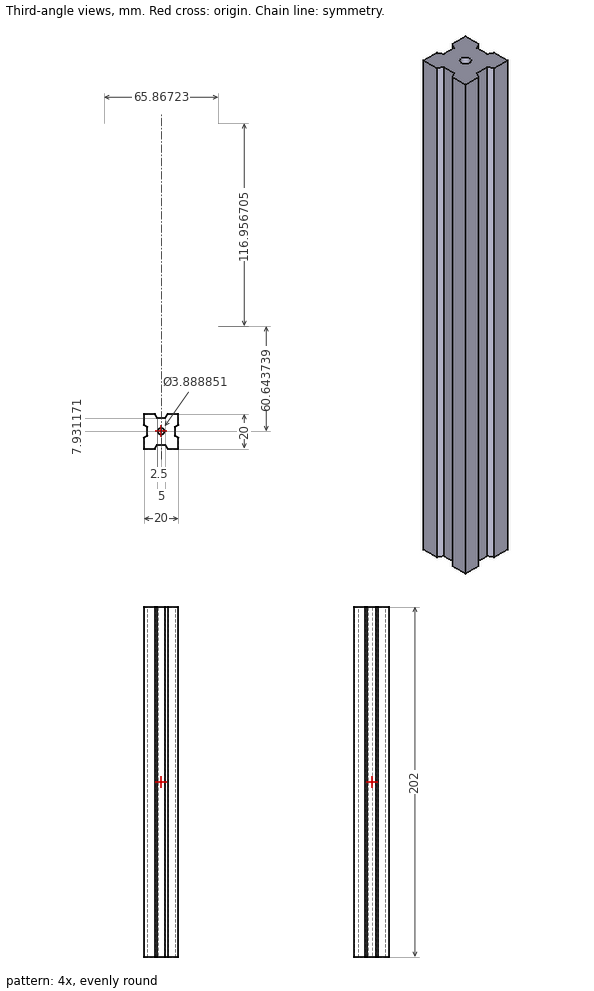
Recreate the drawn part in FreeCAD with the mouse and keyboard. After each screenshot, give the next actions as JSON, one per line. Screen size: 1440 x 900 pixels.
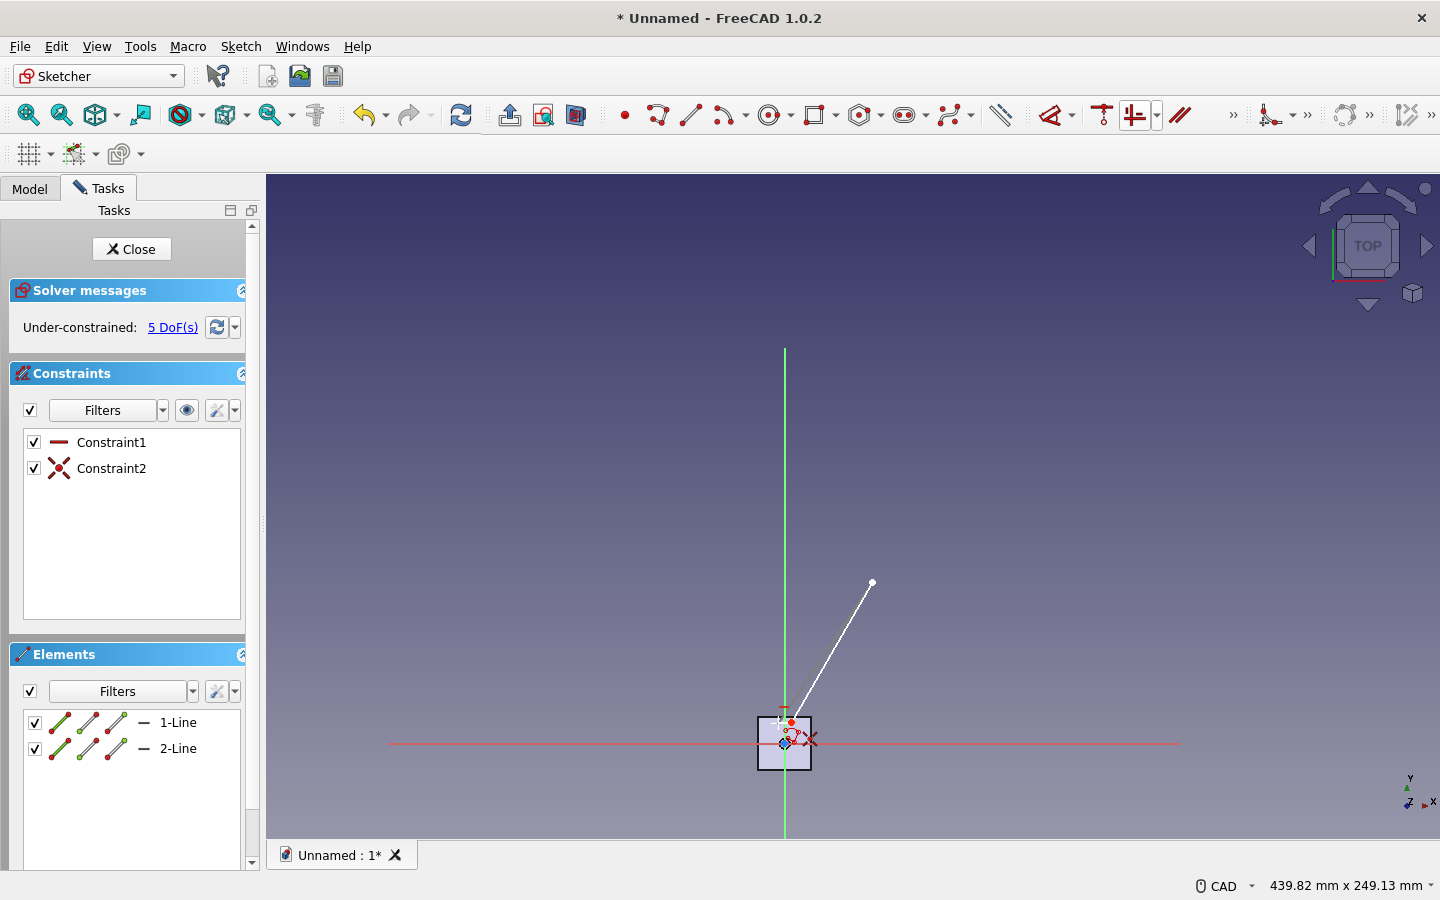
{"action": "left_click", "coordinate": [873, 270]}
{"action": "left_click", "coordinate": [697, 270]}
{"action": "left_click", "coordinate": [697, 582]}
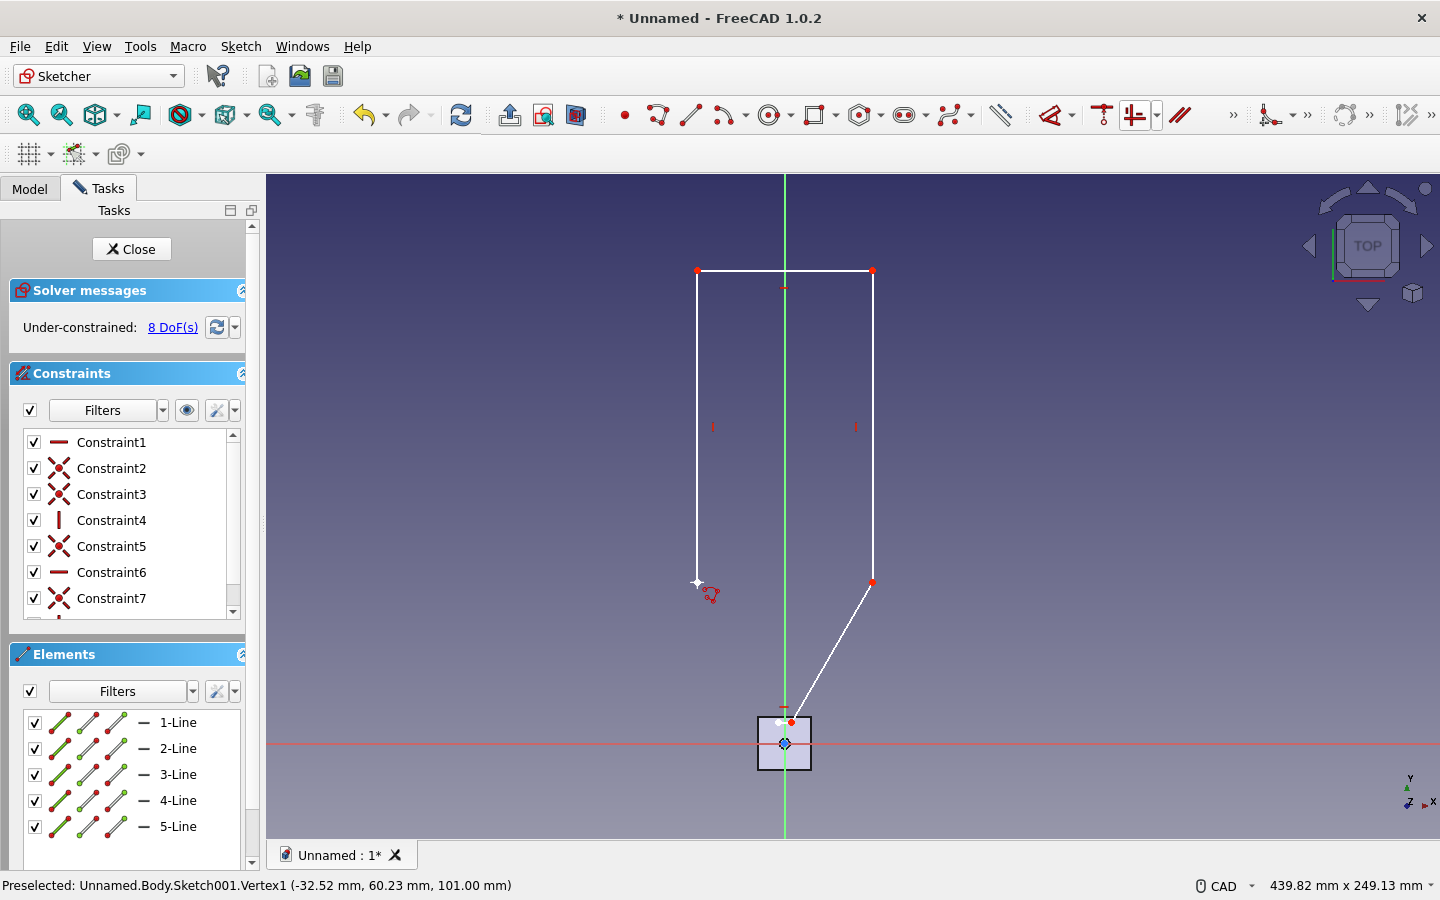
{"action": "scroll", "coordinate": [778, 723], "scroll_direction": "up", "scroll_amount": 5}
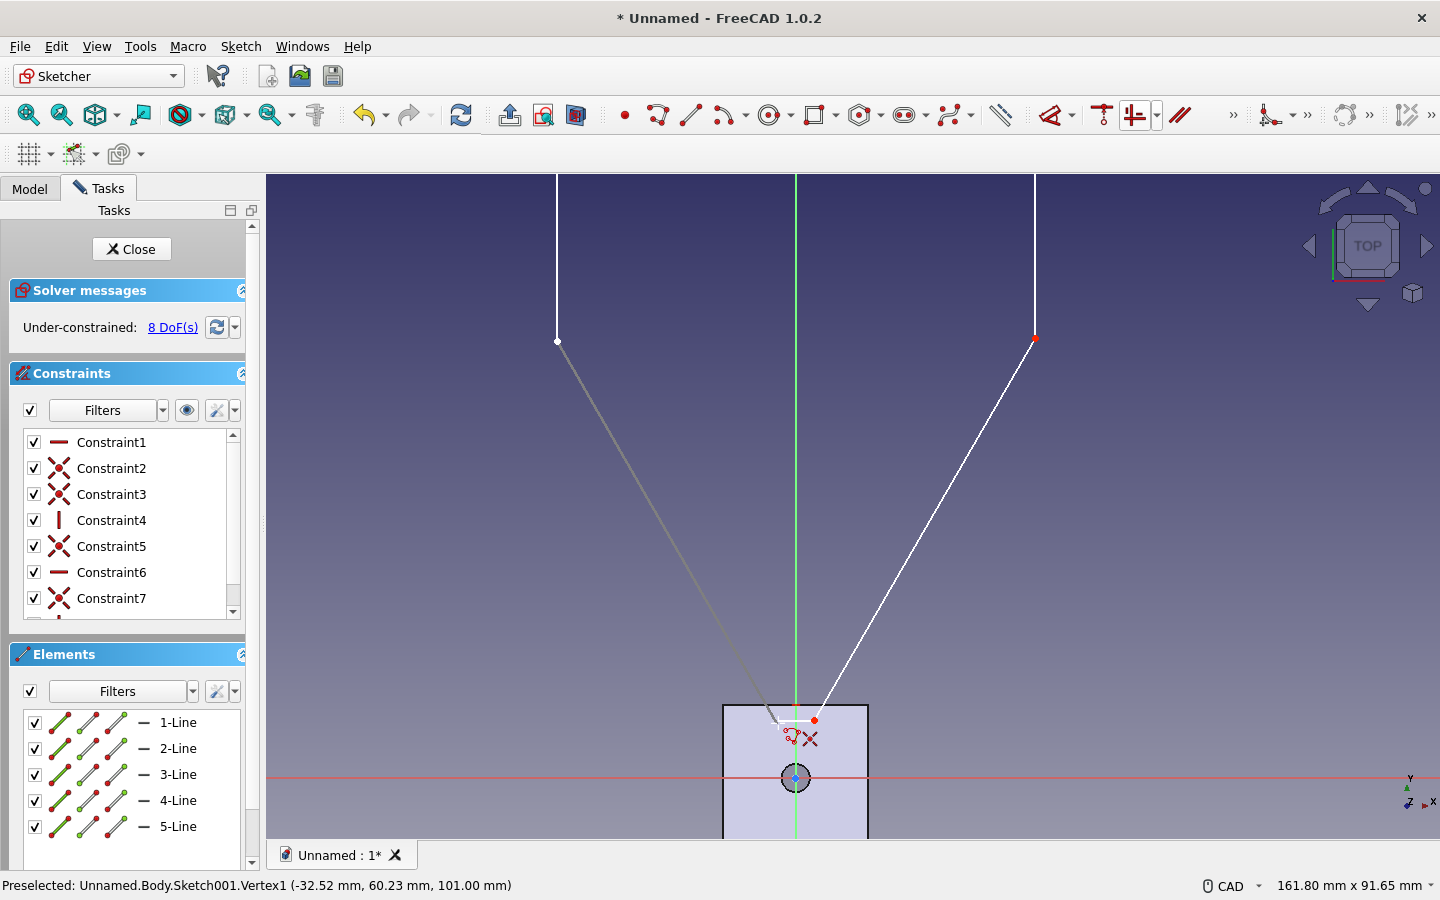
{"action": "left_click", "coordinate": [778, 721]}
{"action": "key", "text": "Escape"}
{"action": "key", "text": "Escape"}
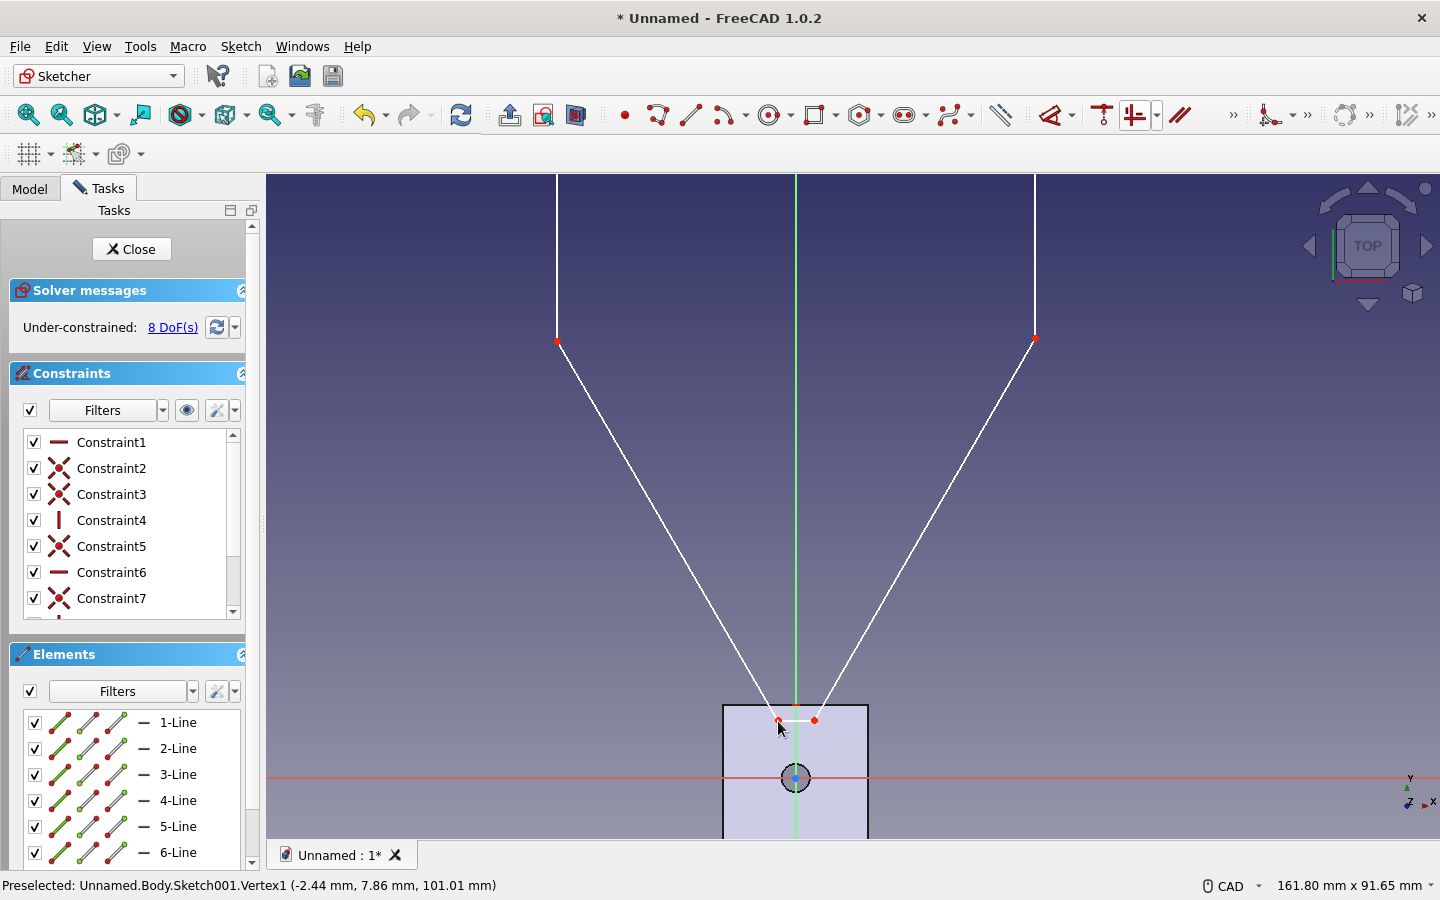
{"action": "left_click", "coordinate": [1035, 339]}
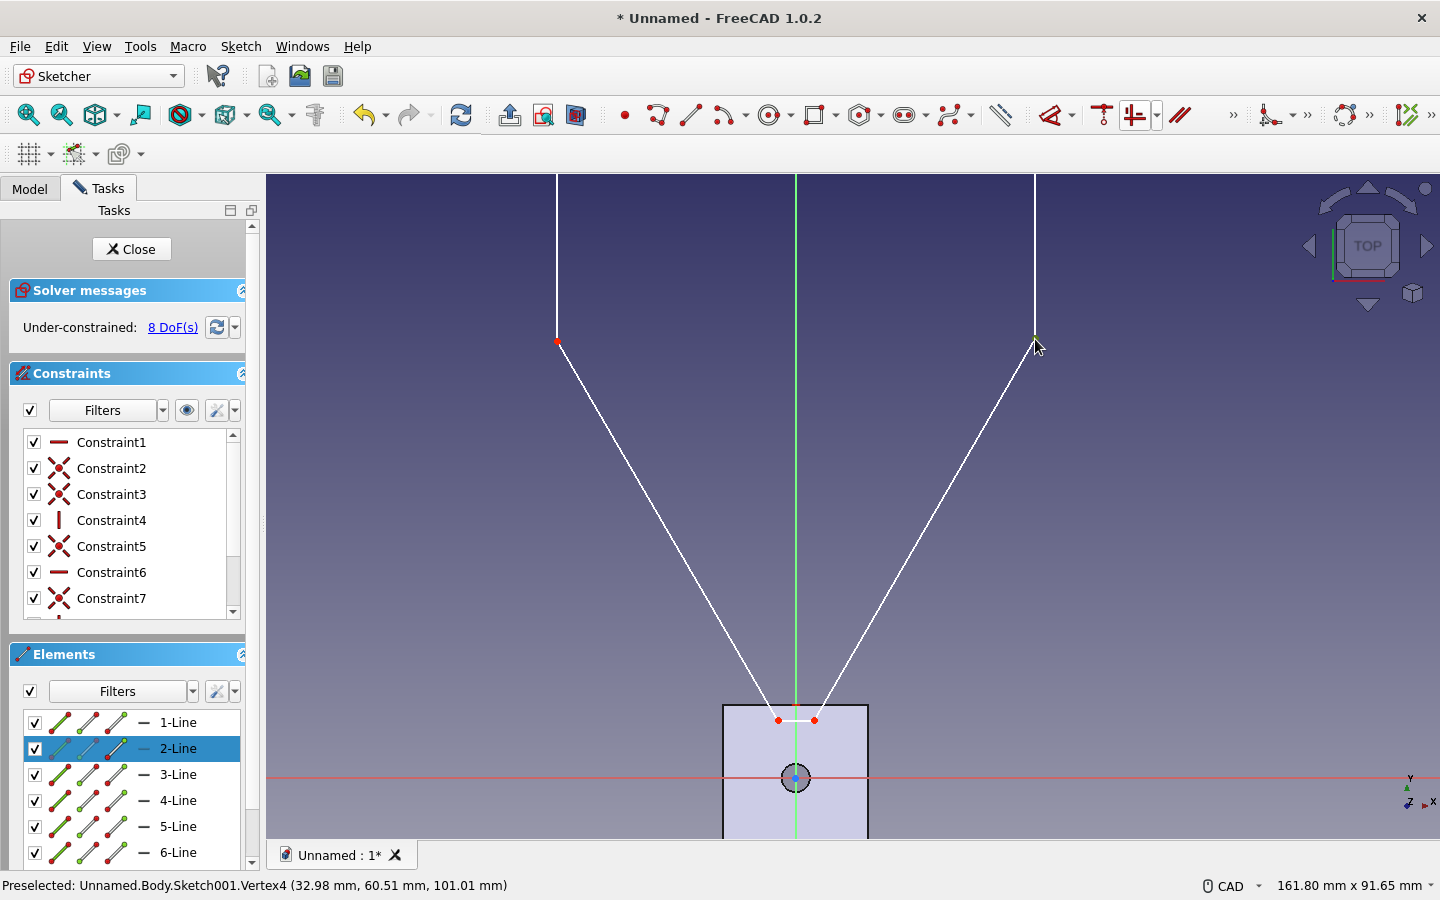
{"action": "left_click", "coordinate": [557, 341]}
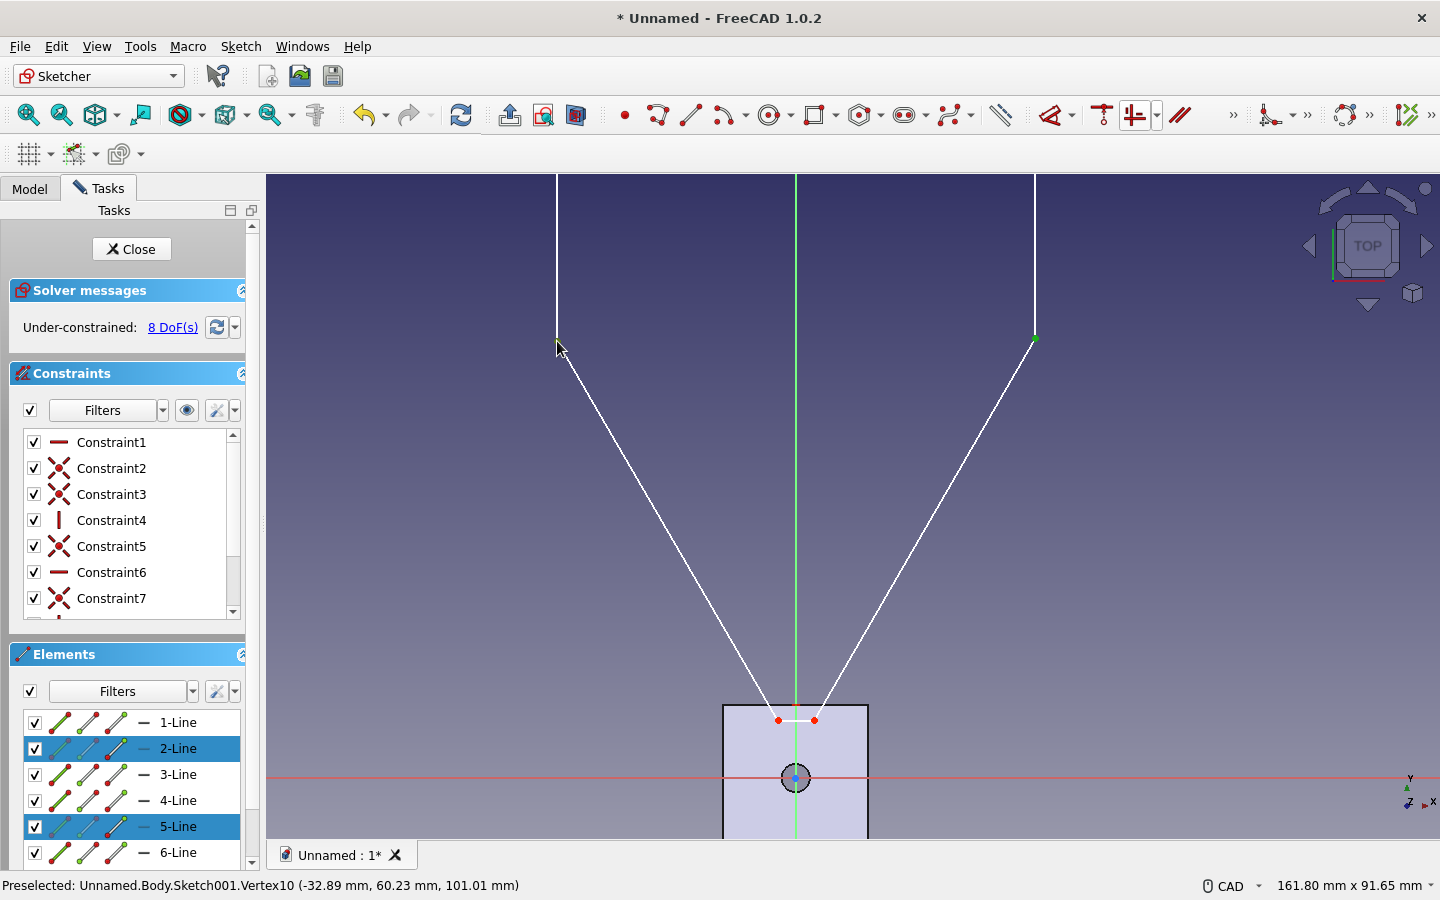
{"action": "left_click", "coordinate": [796, 680]}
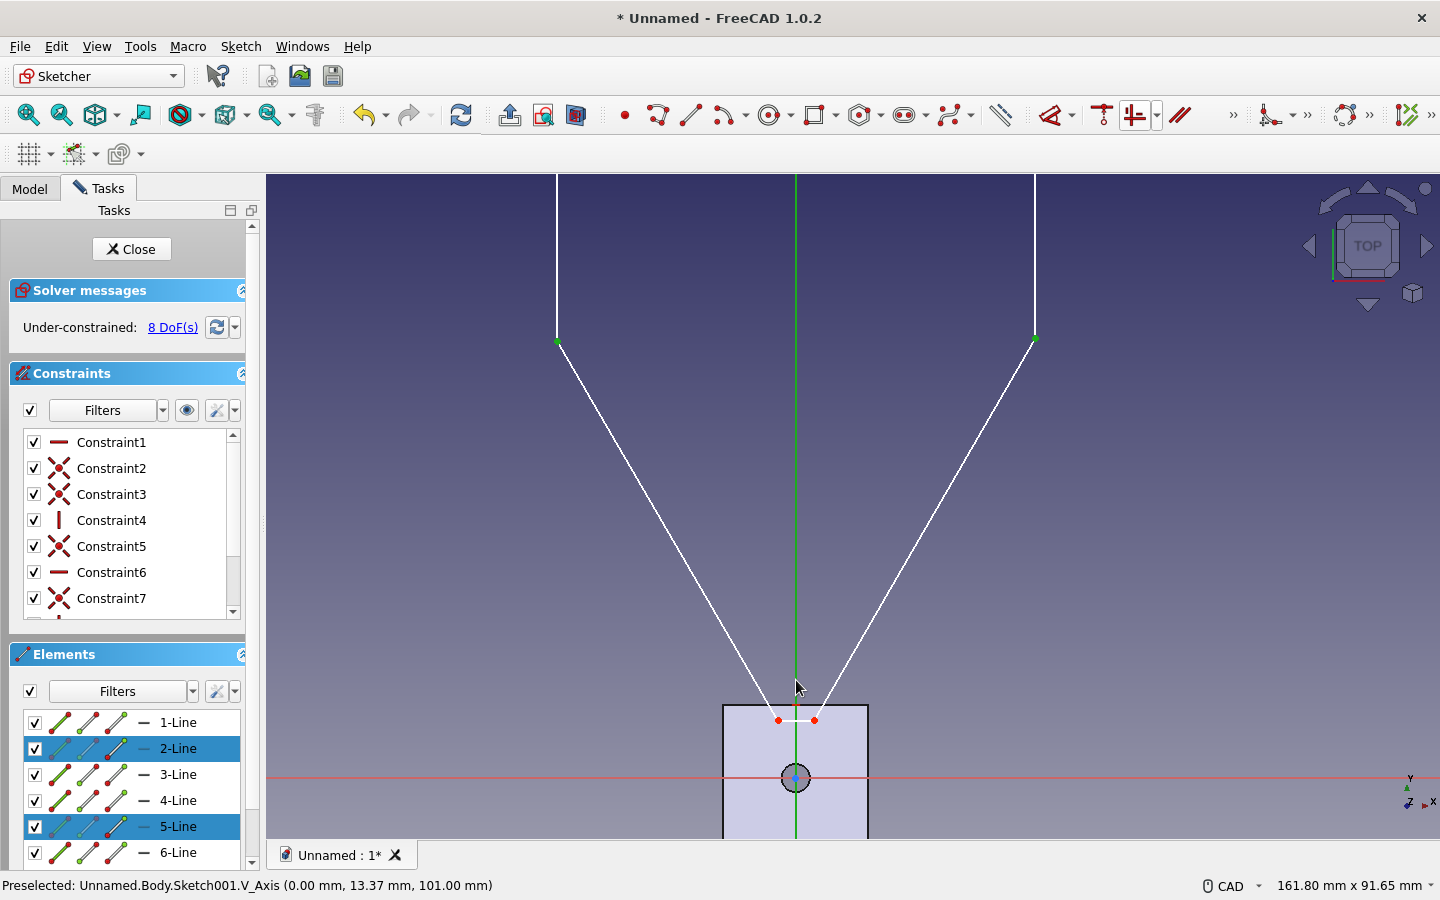
{"action": "key", "text": "s"}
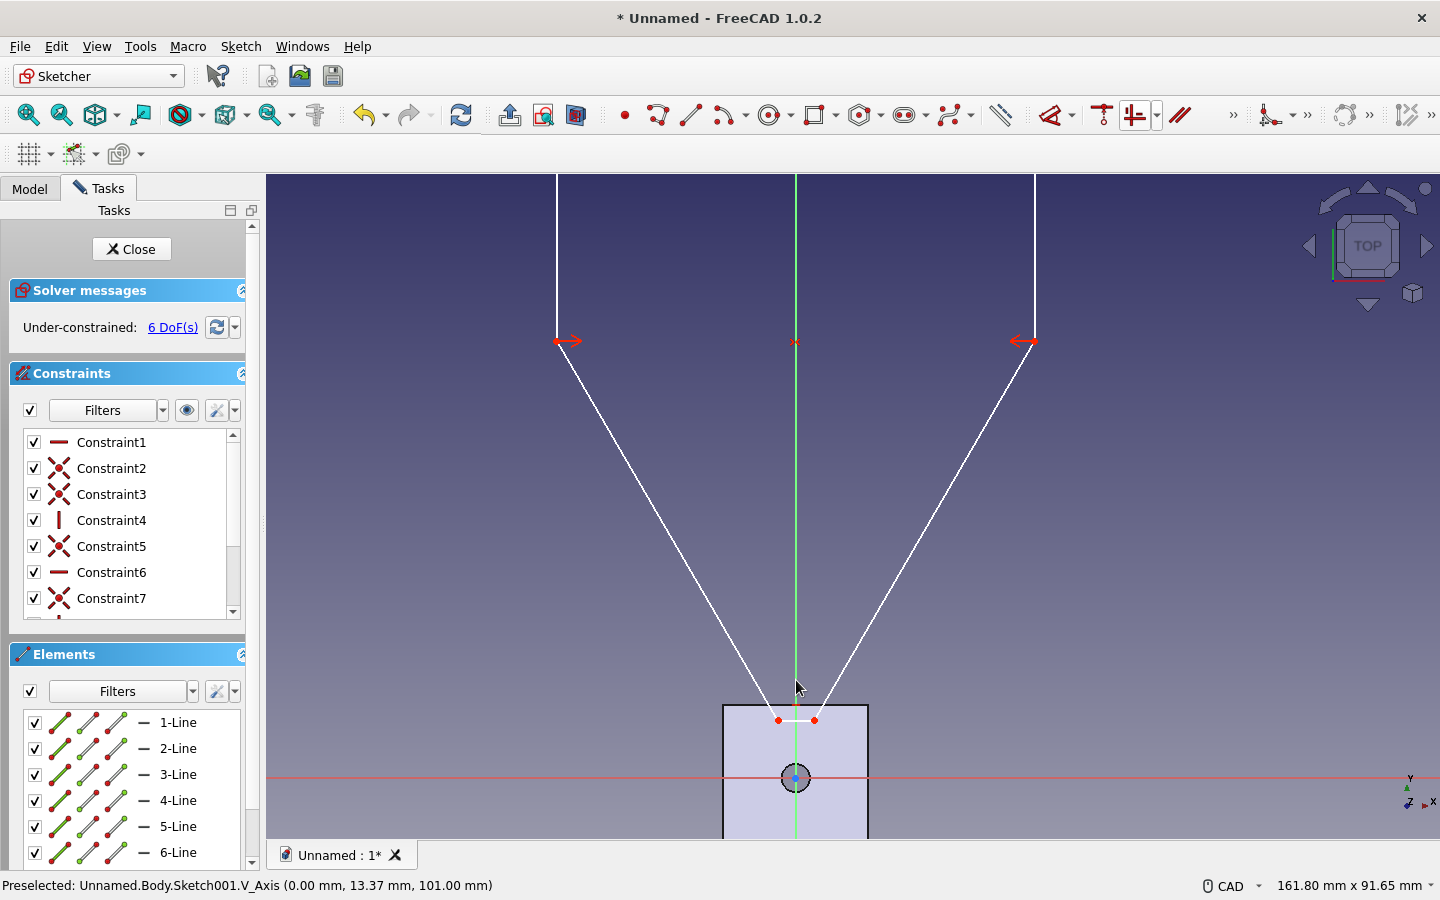
{"action": "left_click", "coordinate": [792, 721]}